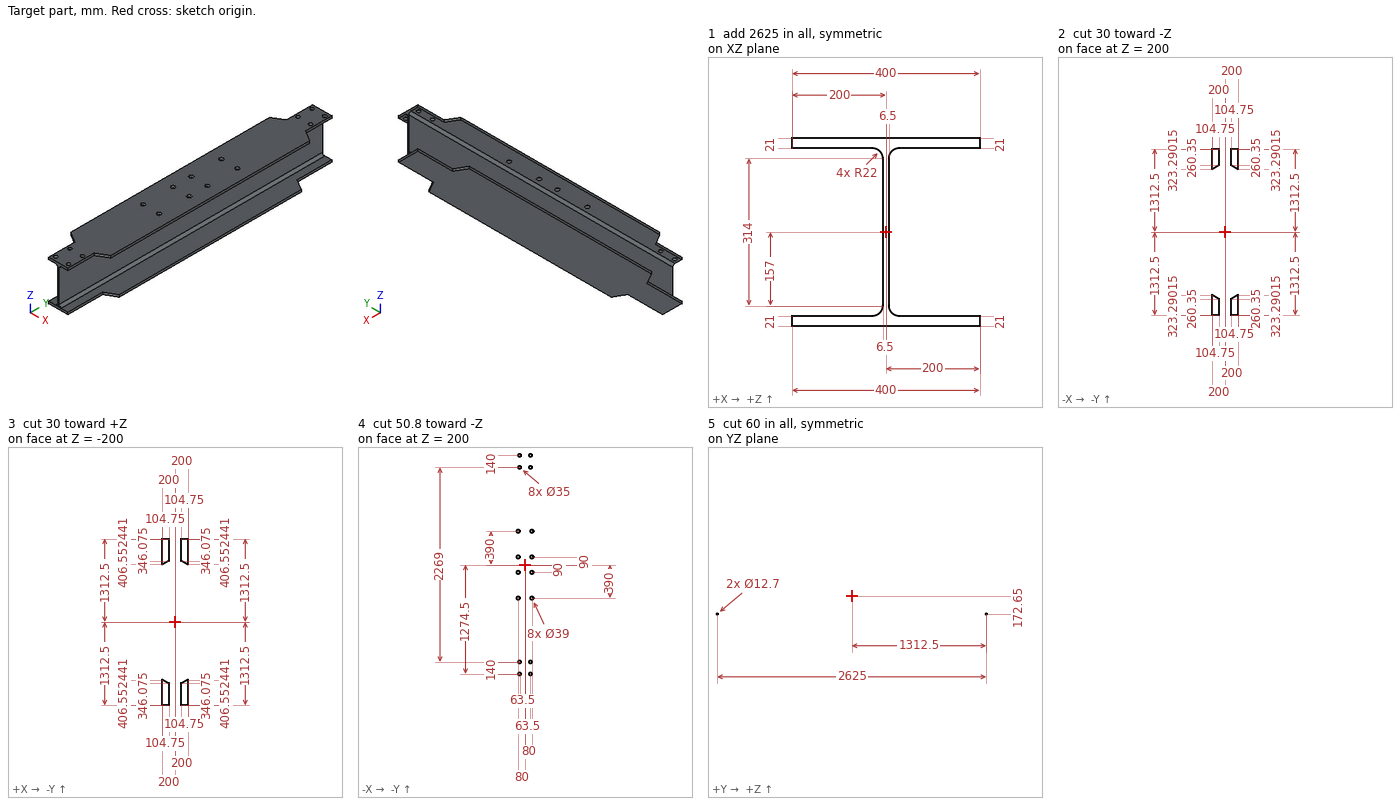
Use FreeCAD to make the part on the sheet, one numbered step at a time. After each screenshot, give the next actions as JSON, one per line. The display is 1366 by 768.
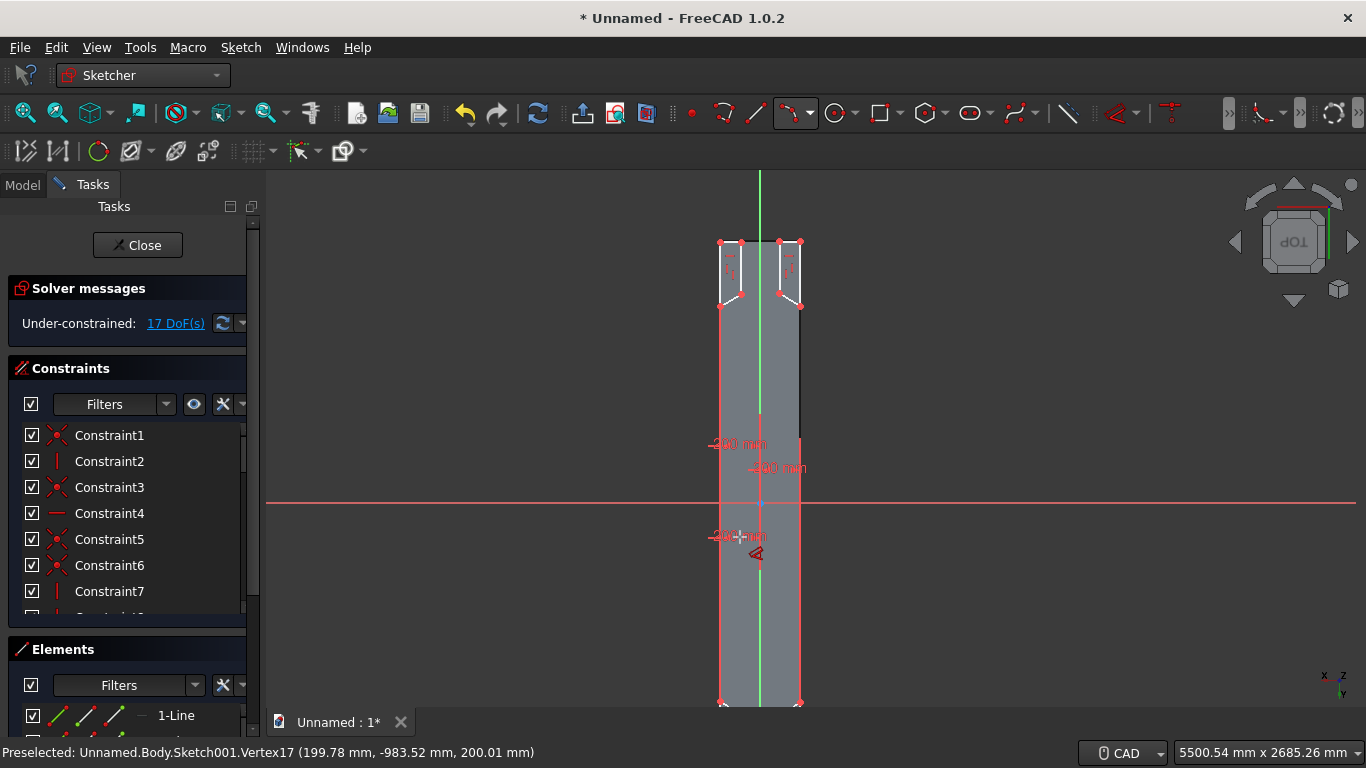
{"action": "left_click", "coordinate": [800, 306]}
{"action": "left_click", "coordinate": [780, 561]}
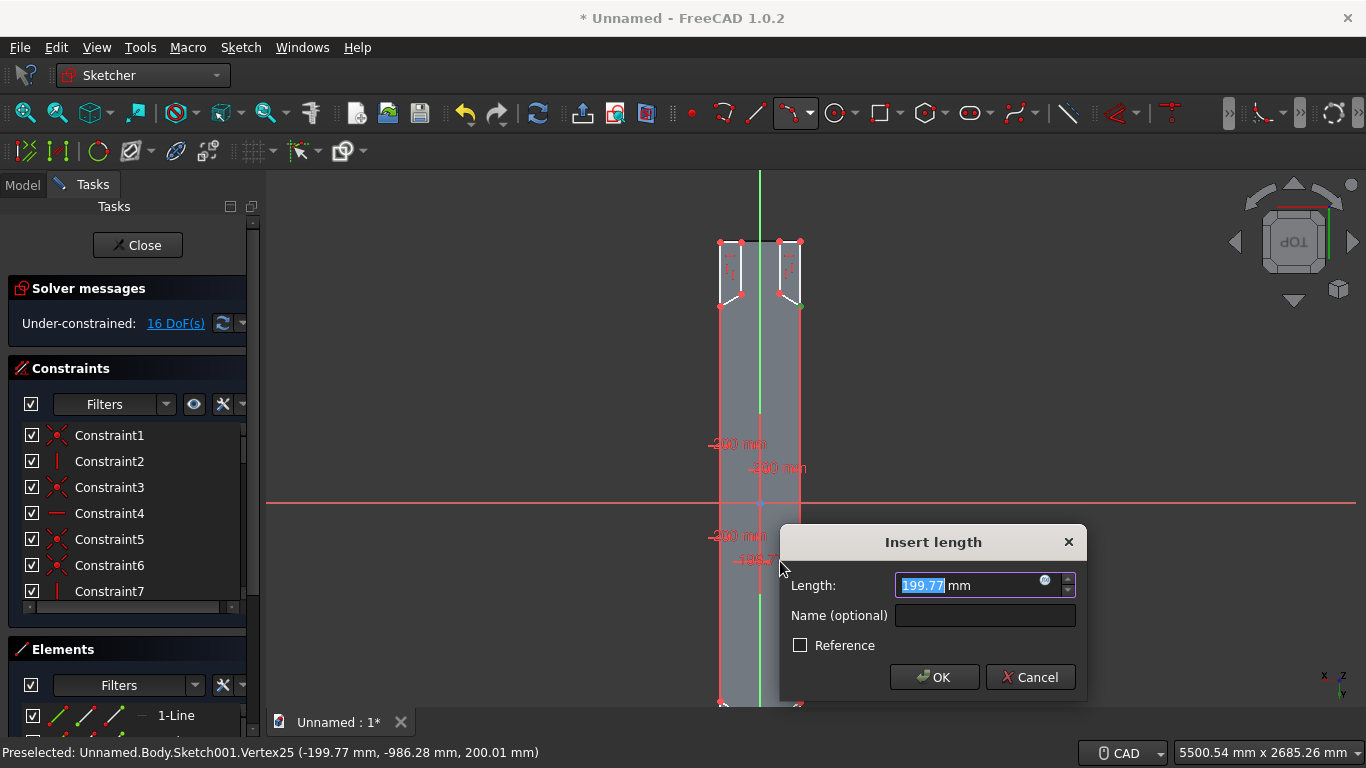
{"action": "type", "text": "200"}
{"action": "key", "text": "Return"}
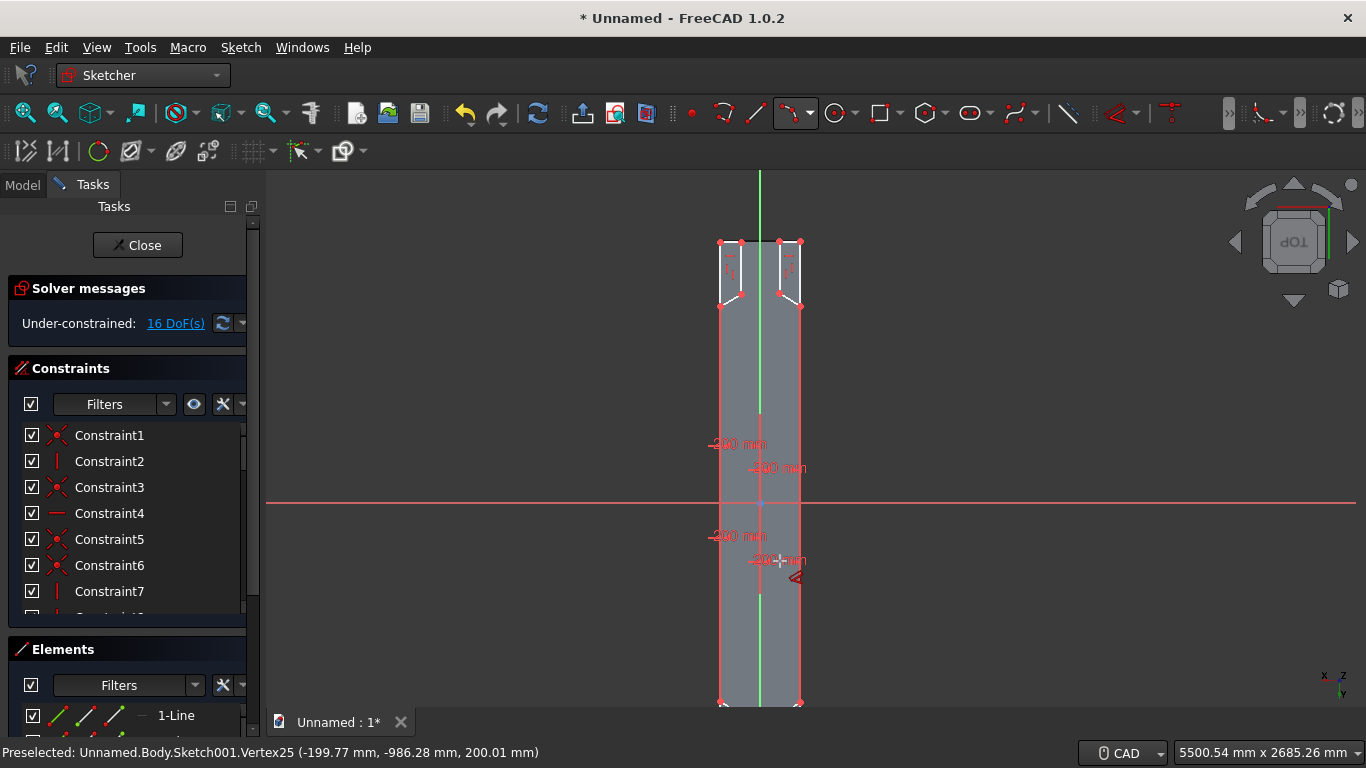
{"action": "scroll", "coordinate": [721, 307], "scroll_direction": "down", "scroll_amount": 2}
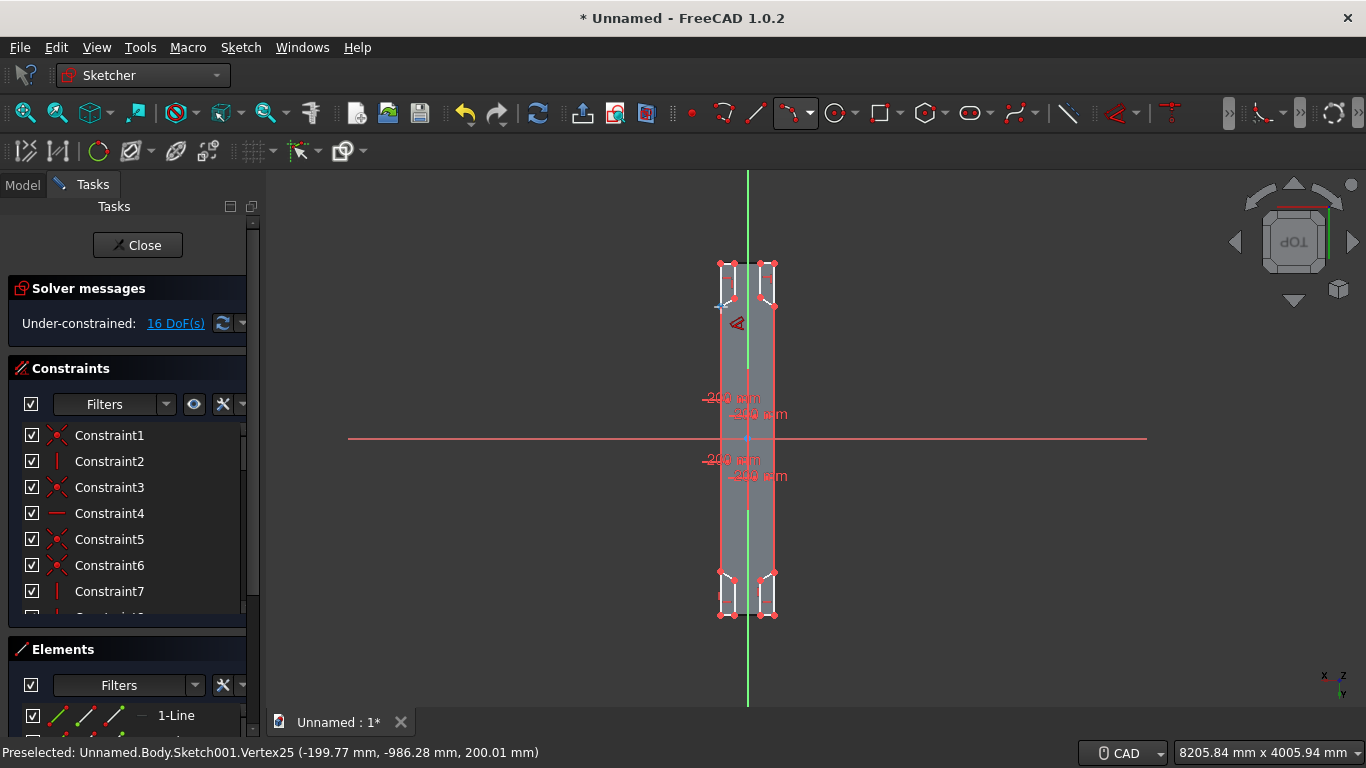
{"action": "scroll", "coordinate": [760, 591], "scroll_direction": "up", "scroll_amount": 2}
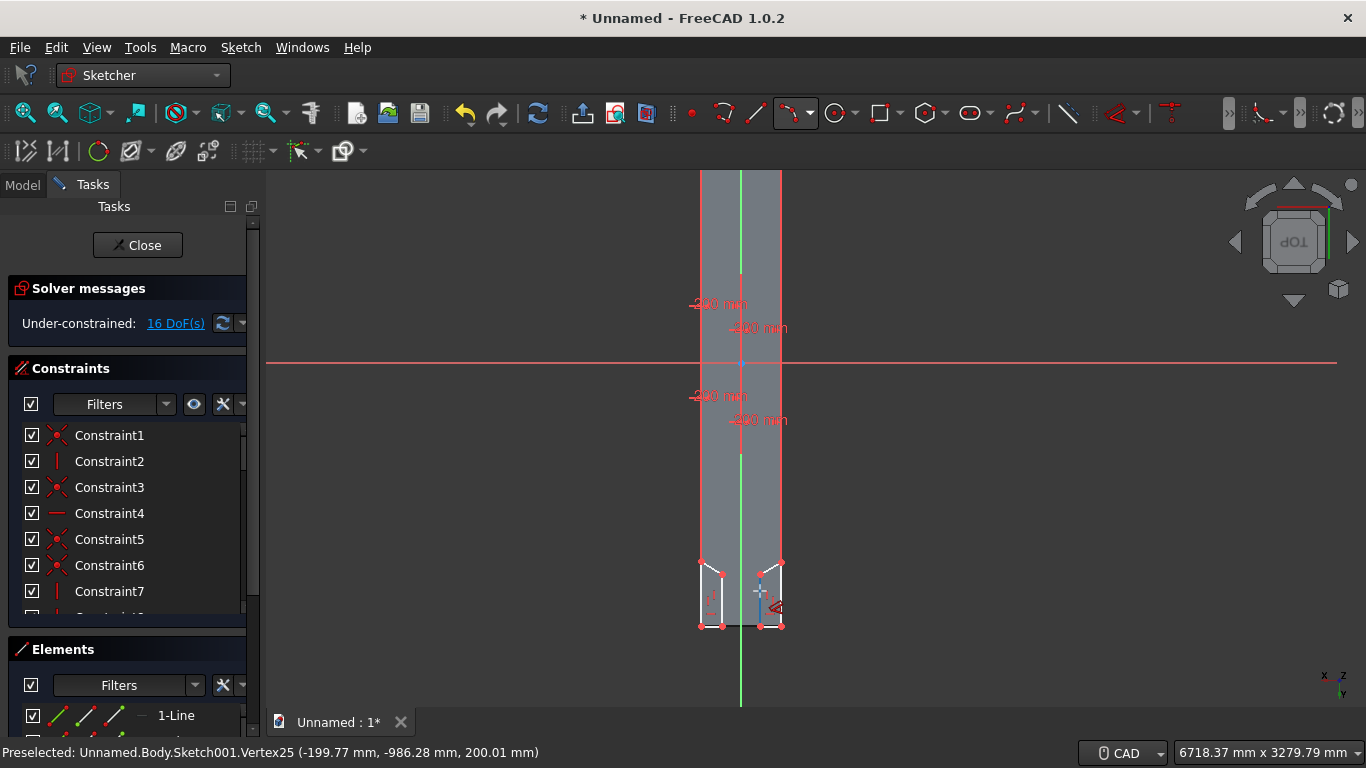
{"action": "left_click", "coordinate": [760, 591]}
{"action": "left_click", "coordinate": [818, 601]}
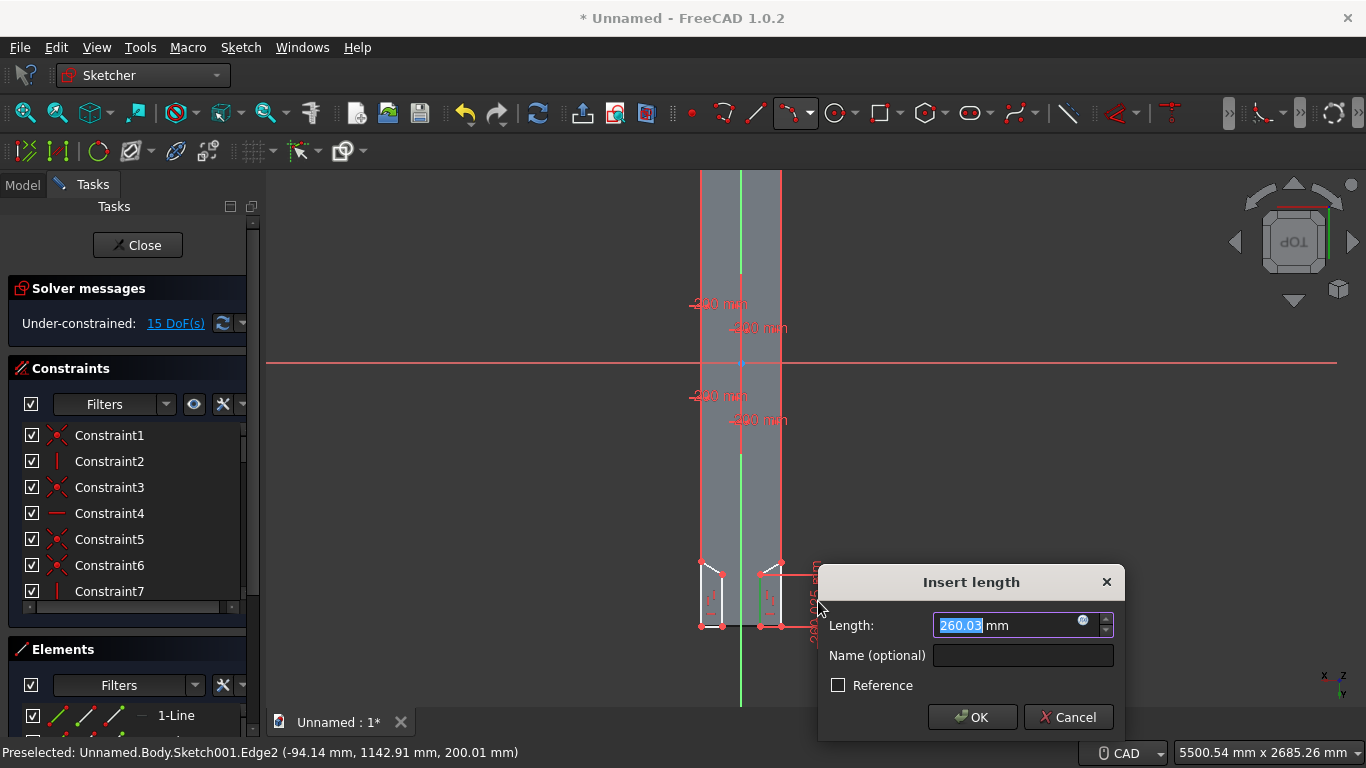
{"action": "type", "text": "260.35"}
{"action": "key", "text": "Return"}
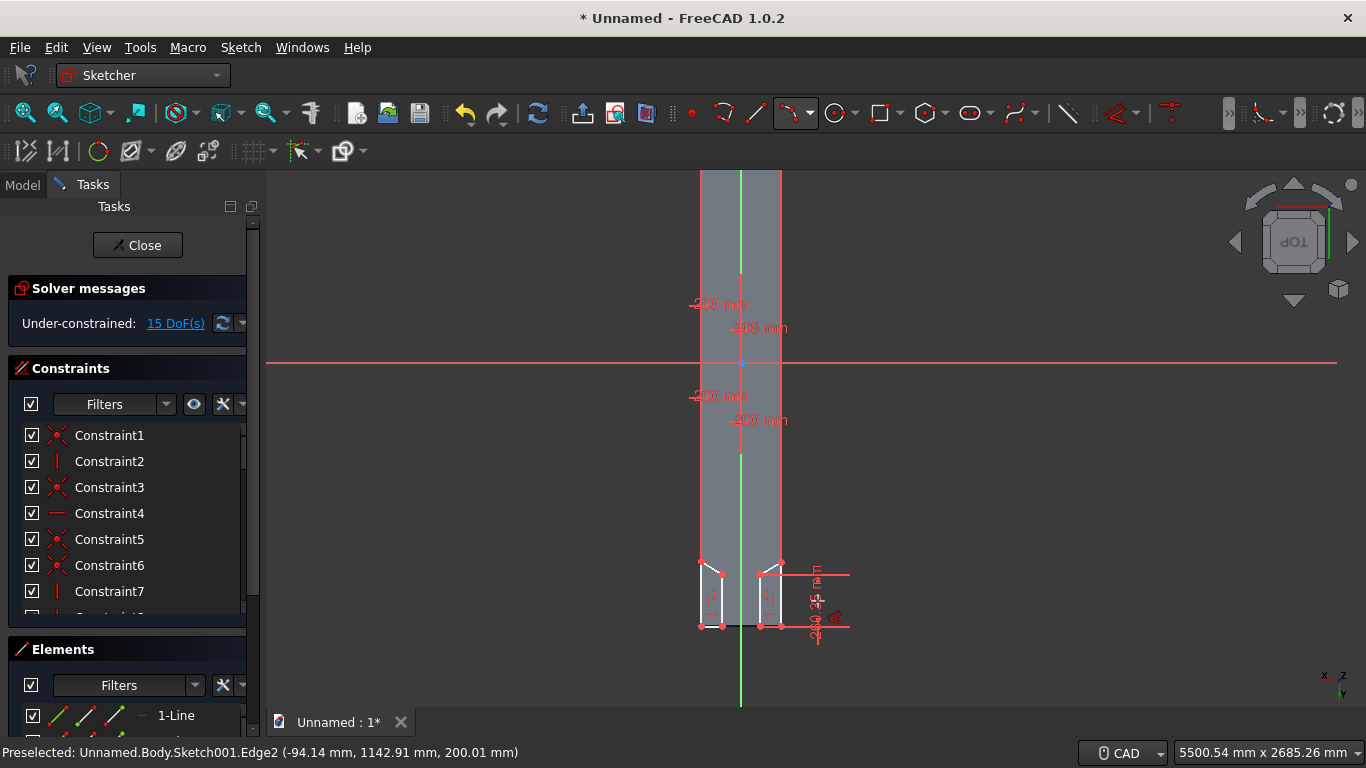
{"action": "scroll", "coordinate": [771, 627], "scroll_direction": "up", "scroll_amount": 4}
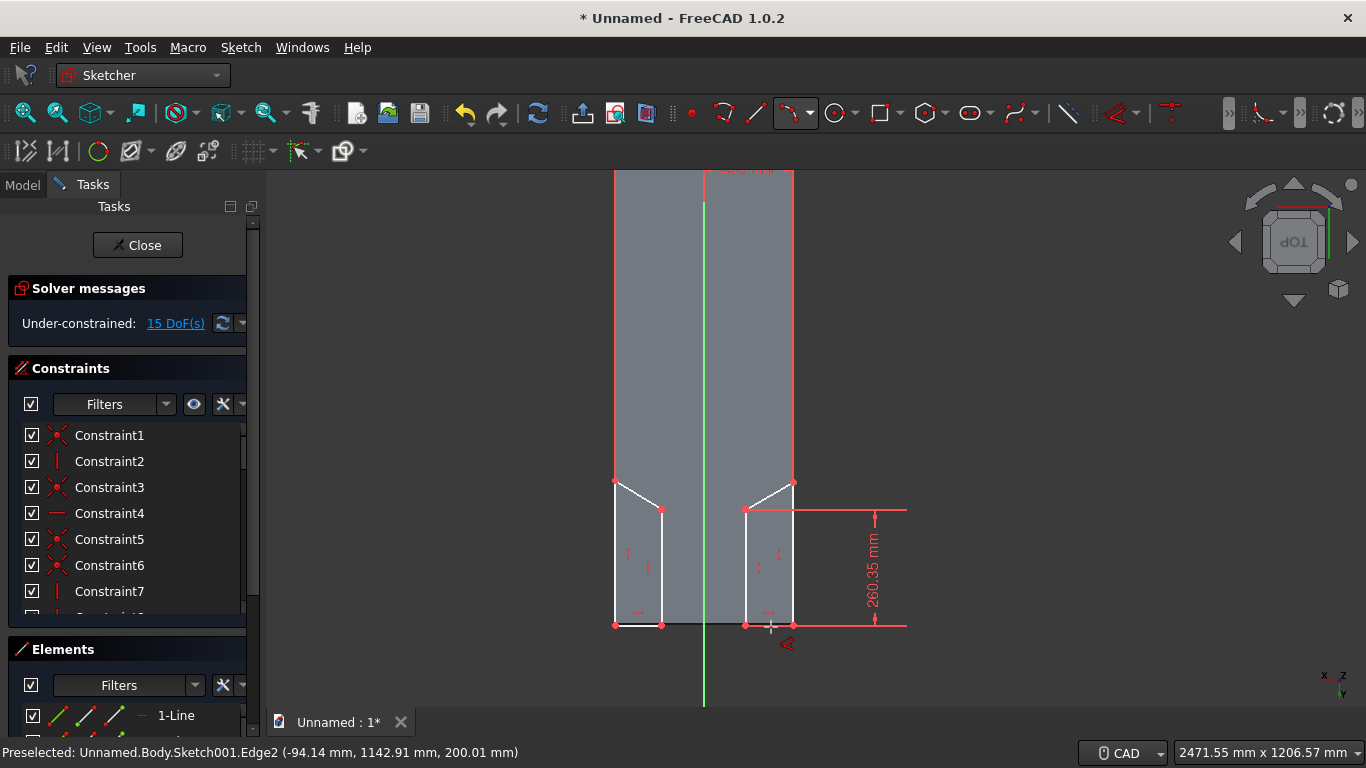
{"action": "left_click", "coordinate": [770, 626]}
{"action": "left_click", "coordinate": [770, 660]}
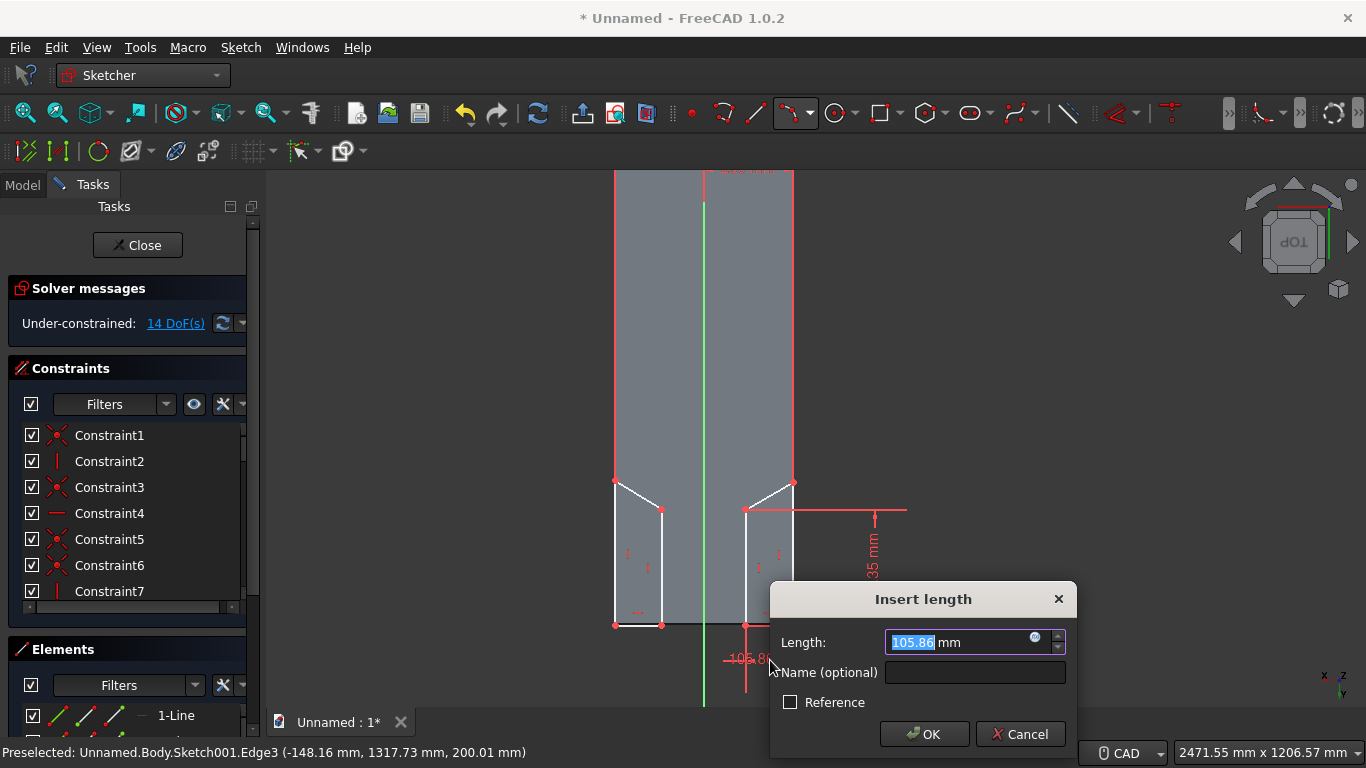
{"action": "type", "text": "104.75"}
{"action": "key", "text": "Return"}